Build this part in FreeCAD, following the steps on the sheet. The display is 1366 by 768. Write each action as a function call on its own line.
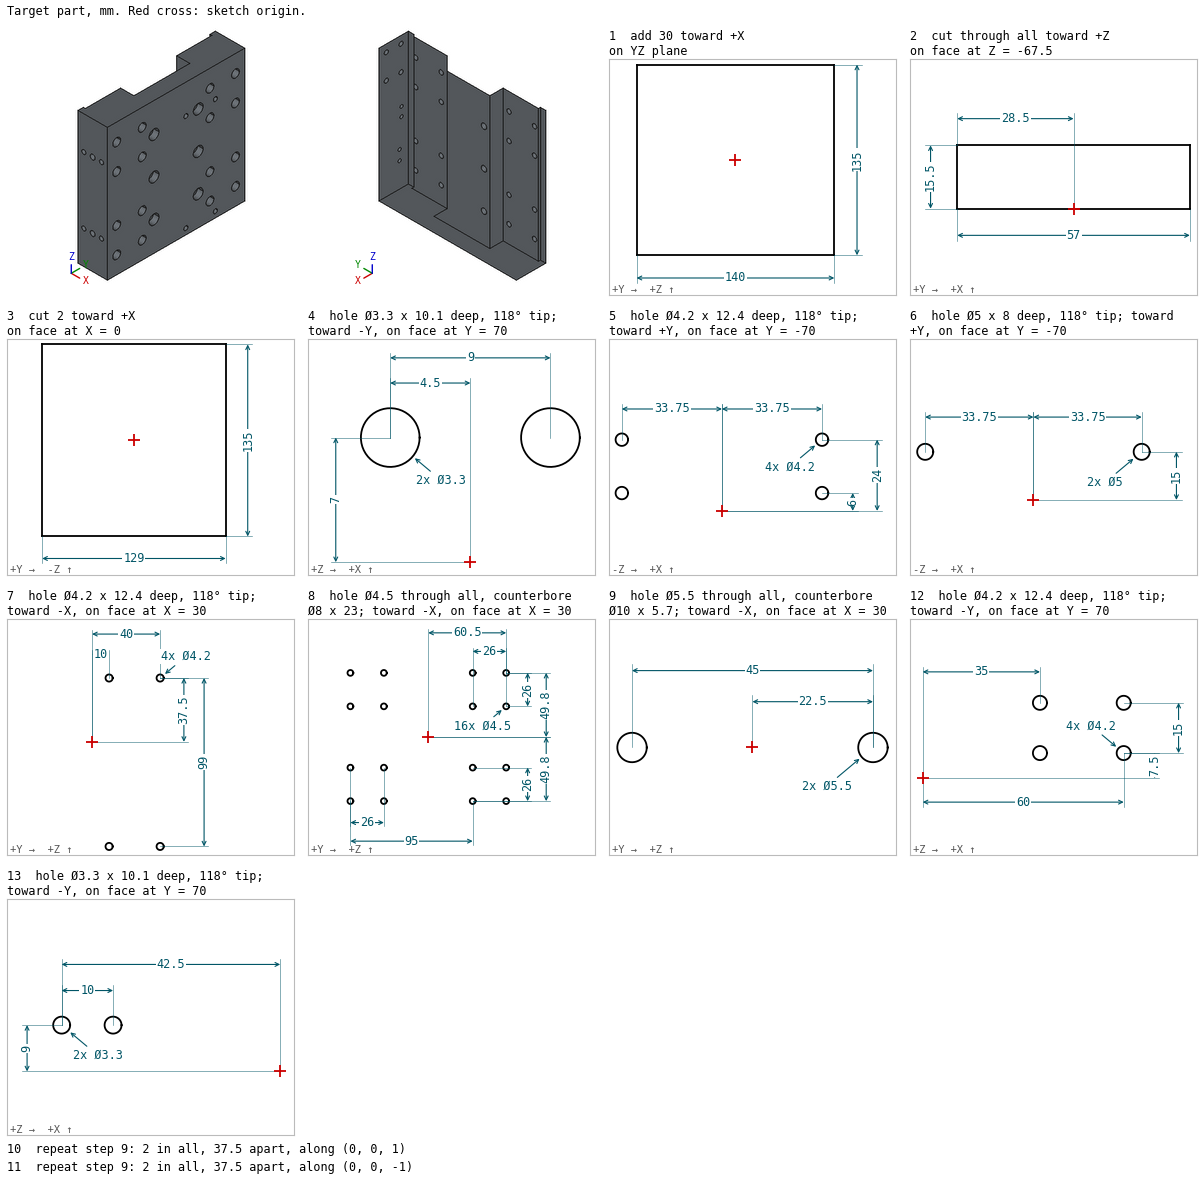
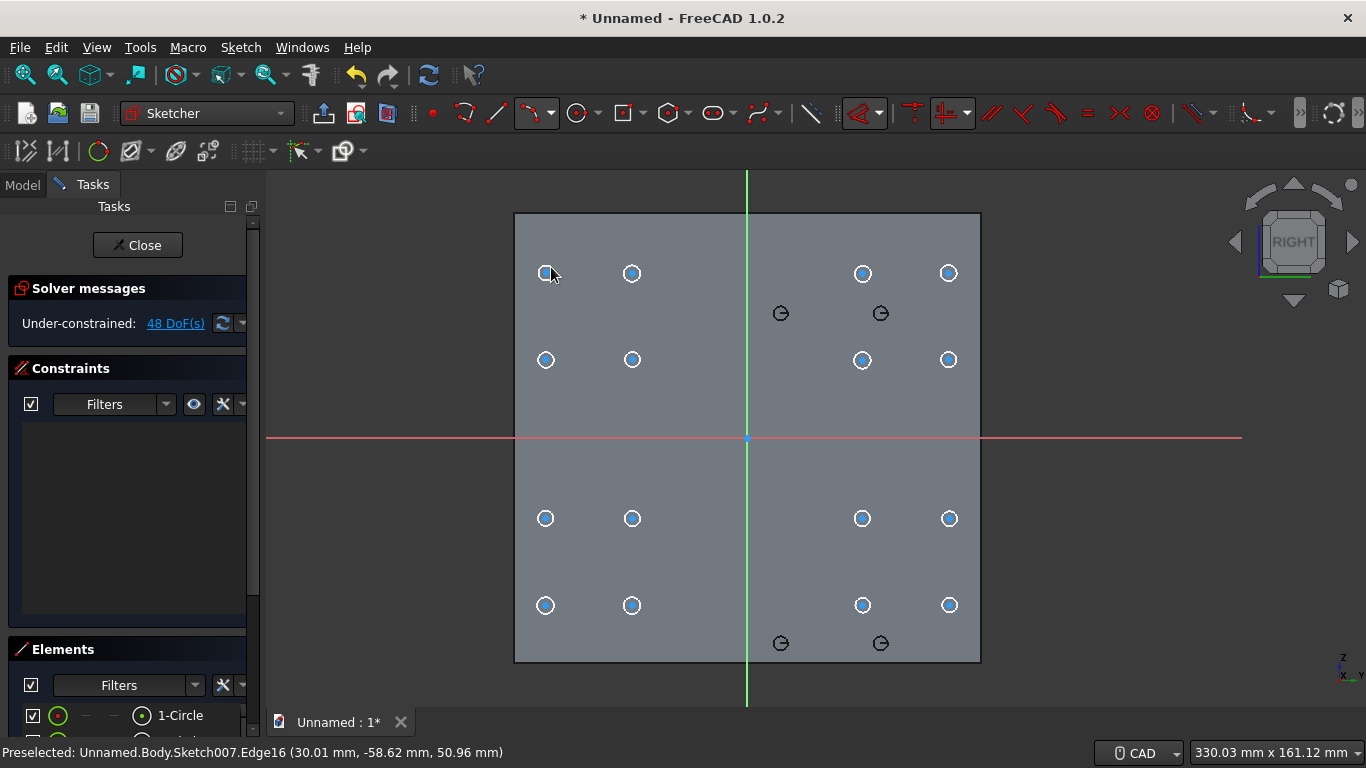
scroll(954, 267, up, 3)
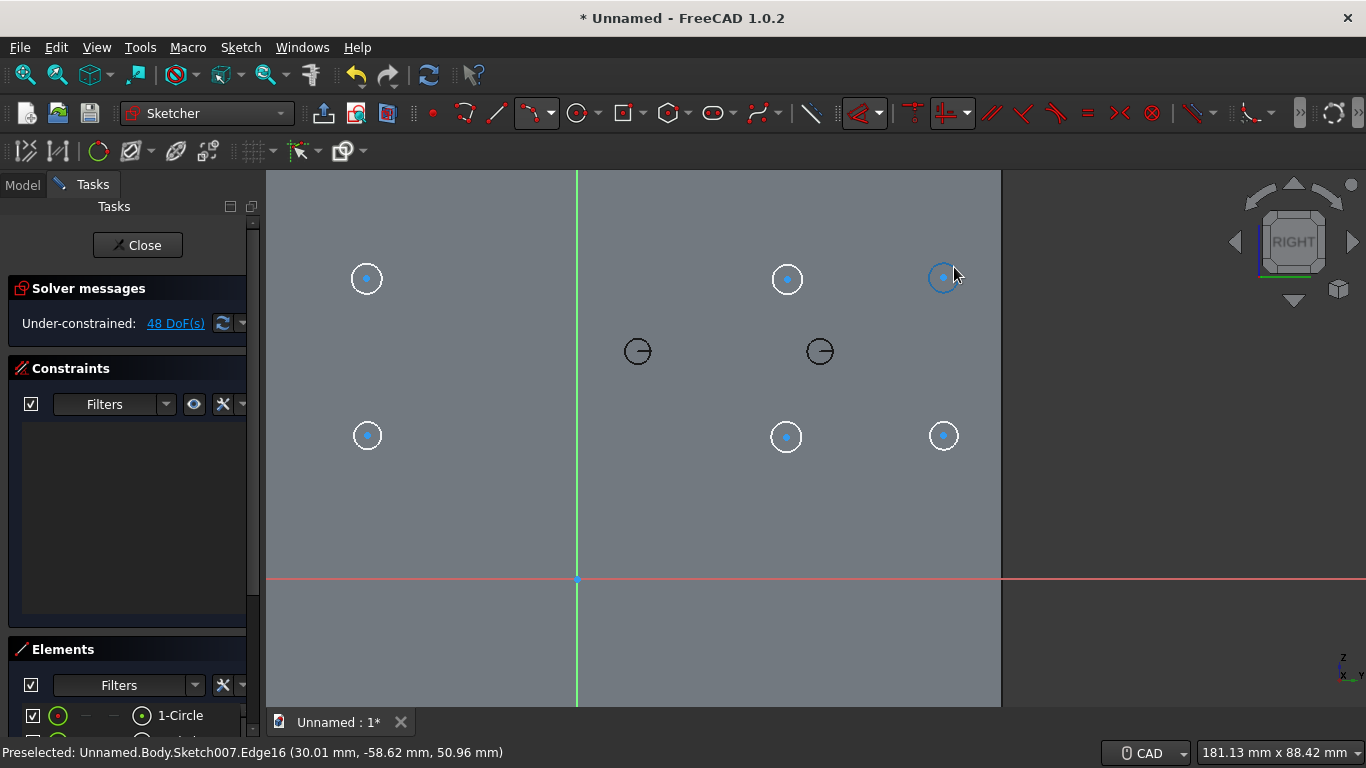
click(954, 268)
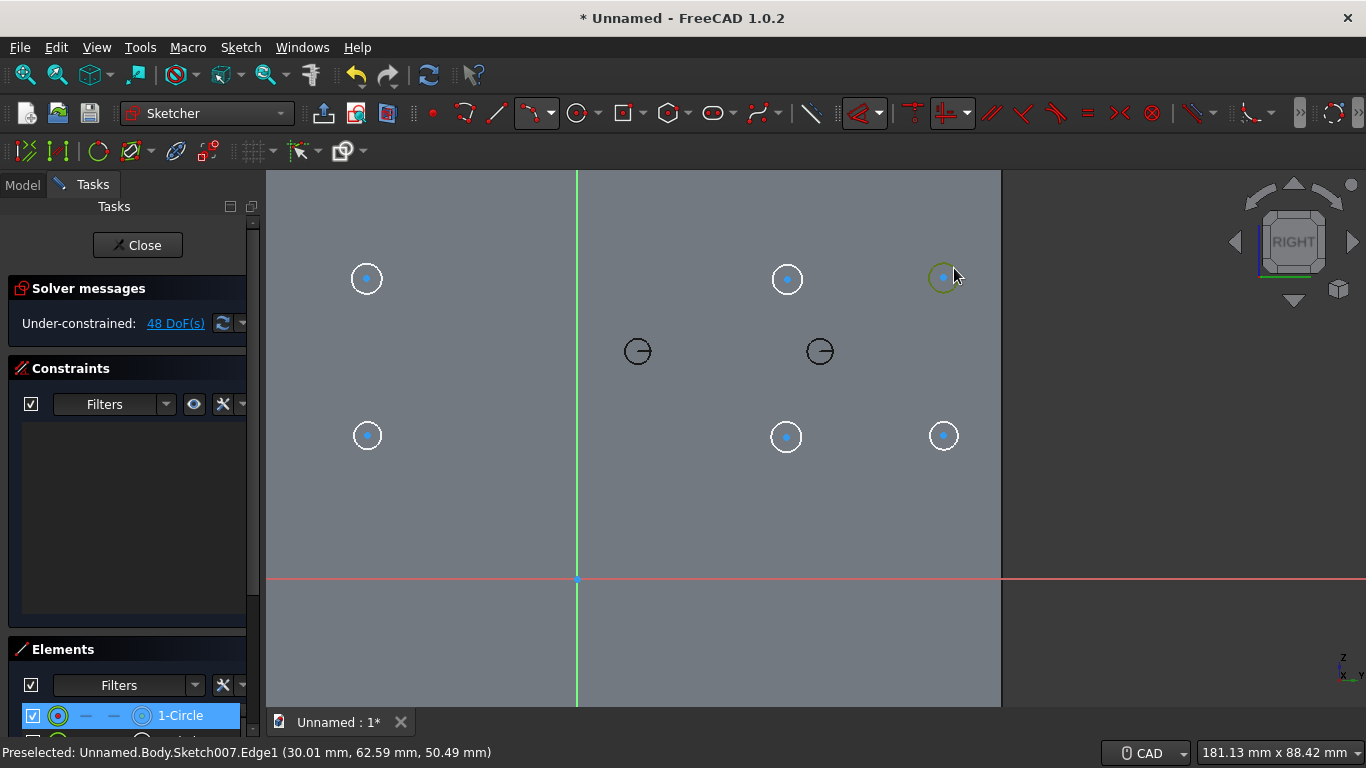
click(954, 426)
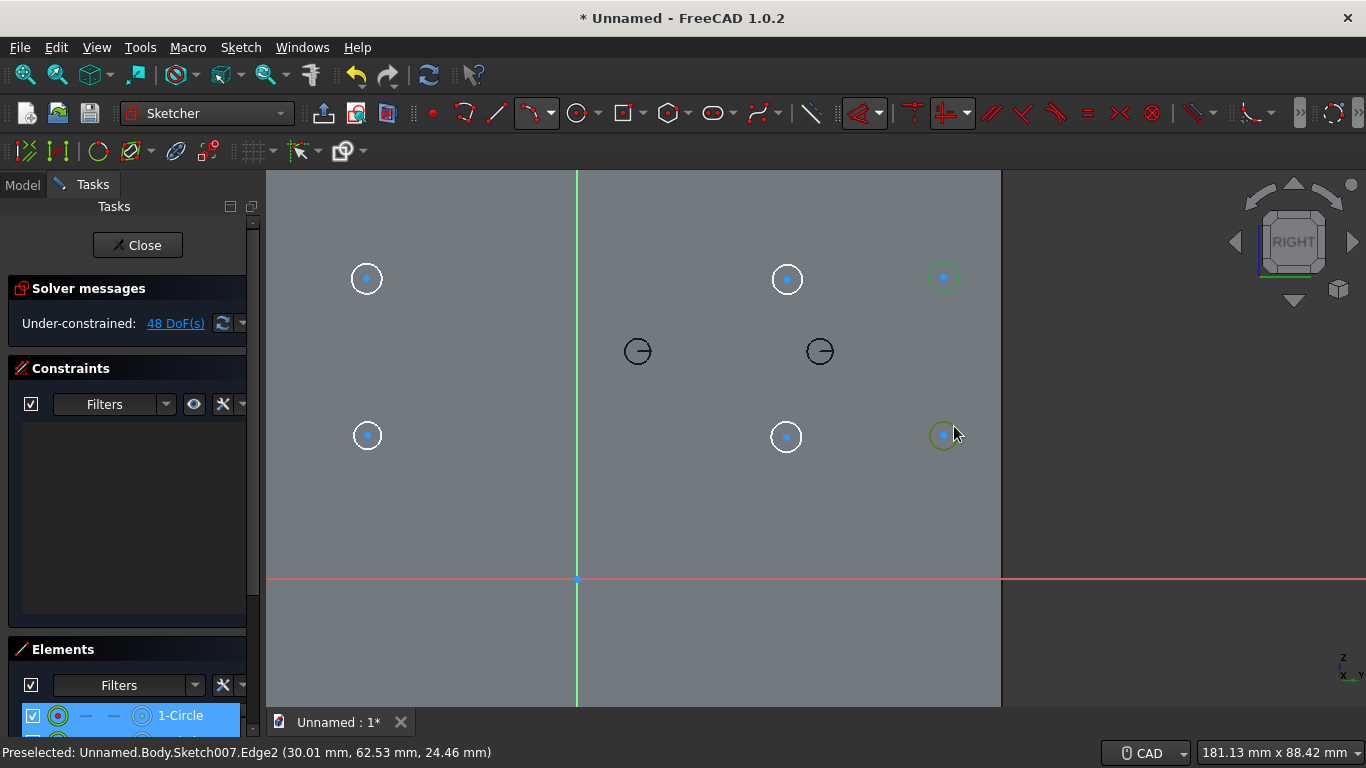
click(797, 426)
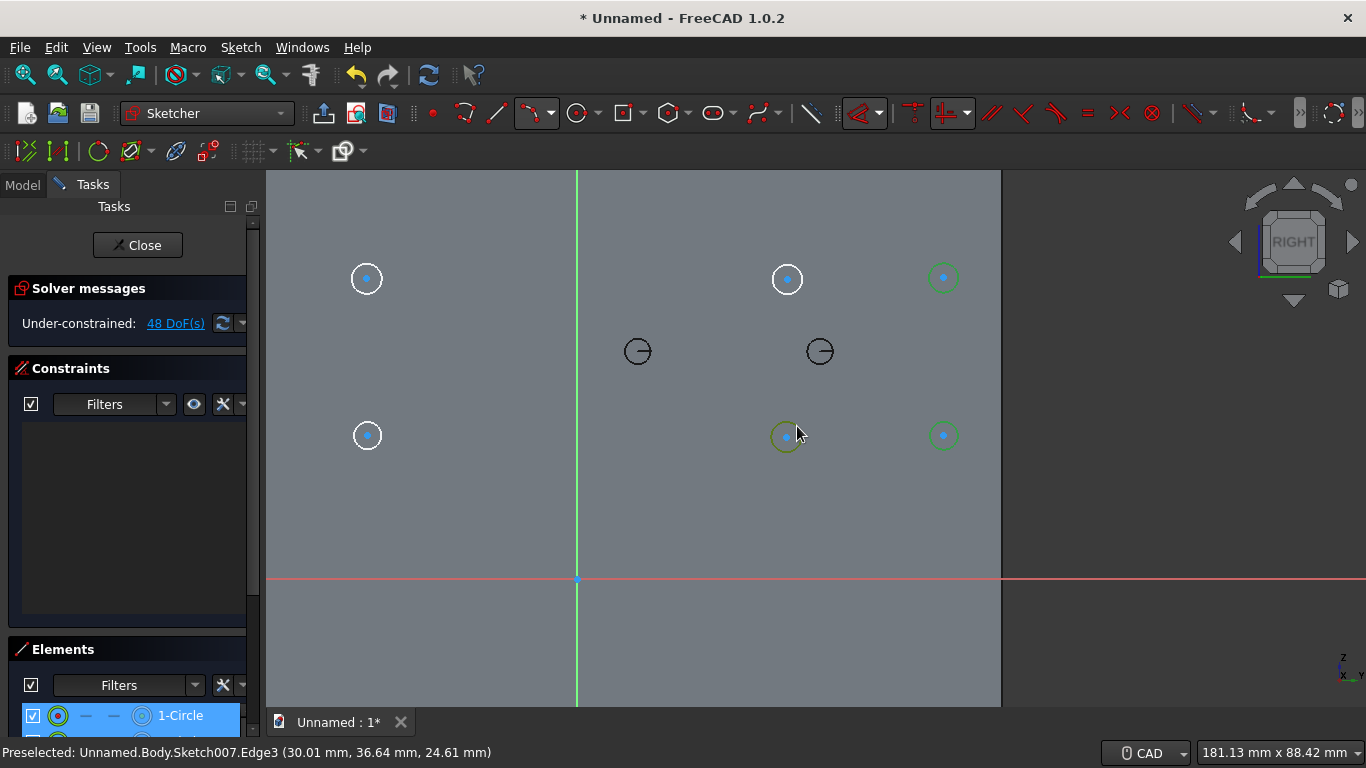
click(798, 269)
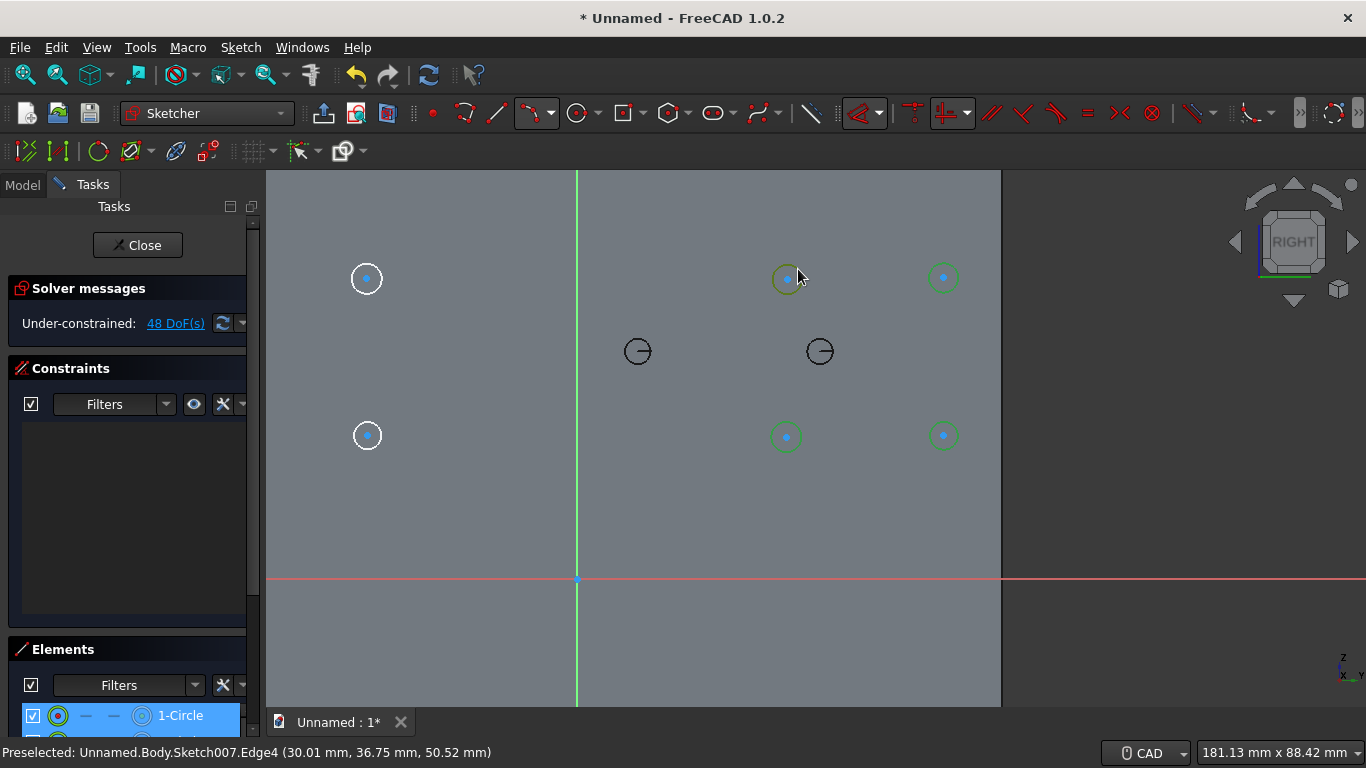
scroll(955, 267, down, 3)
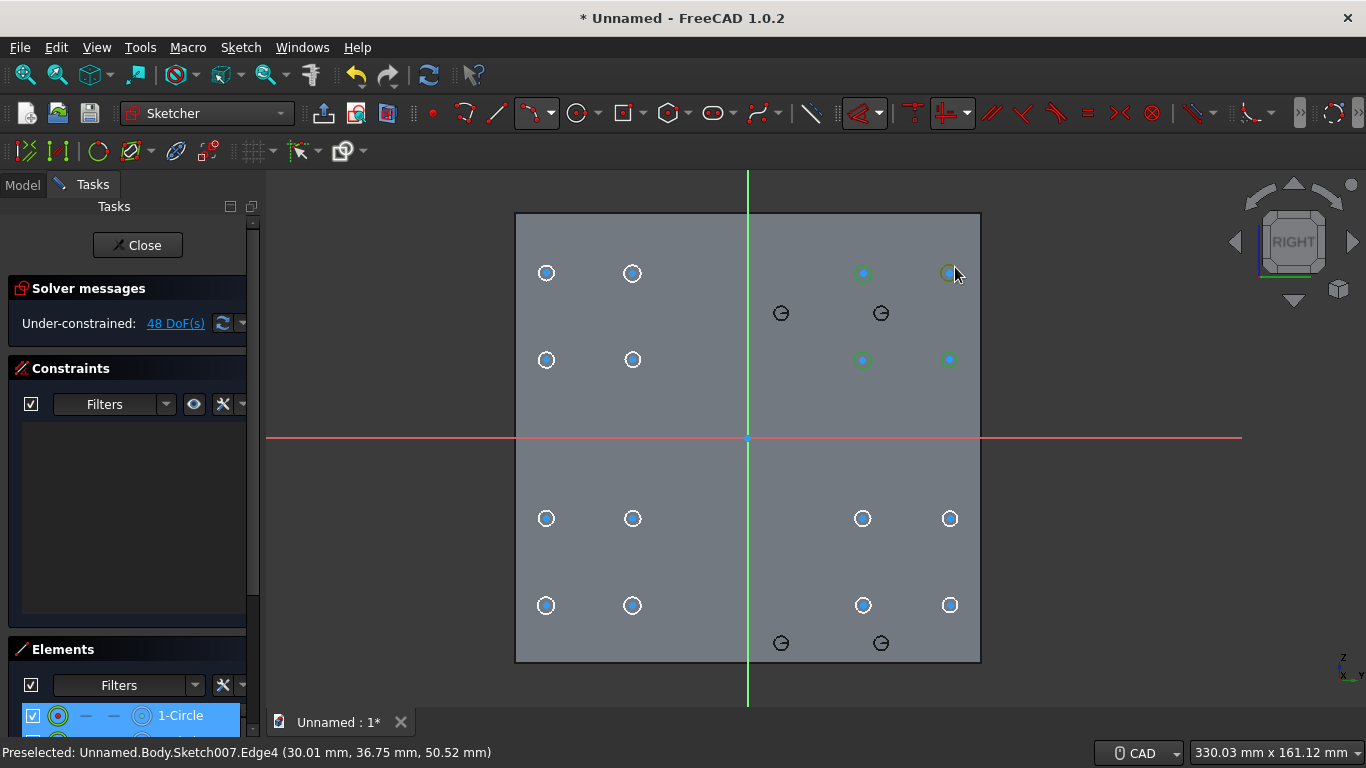
scroll(868, 600, up, 4)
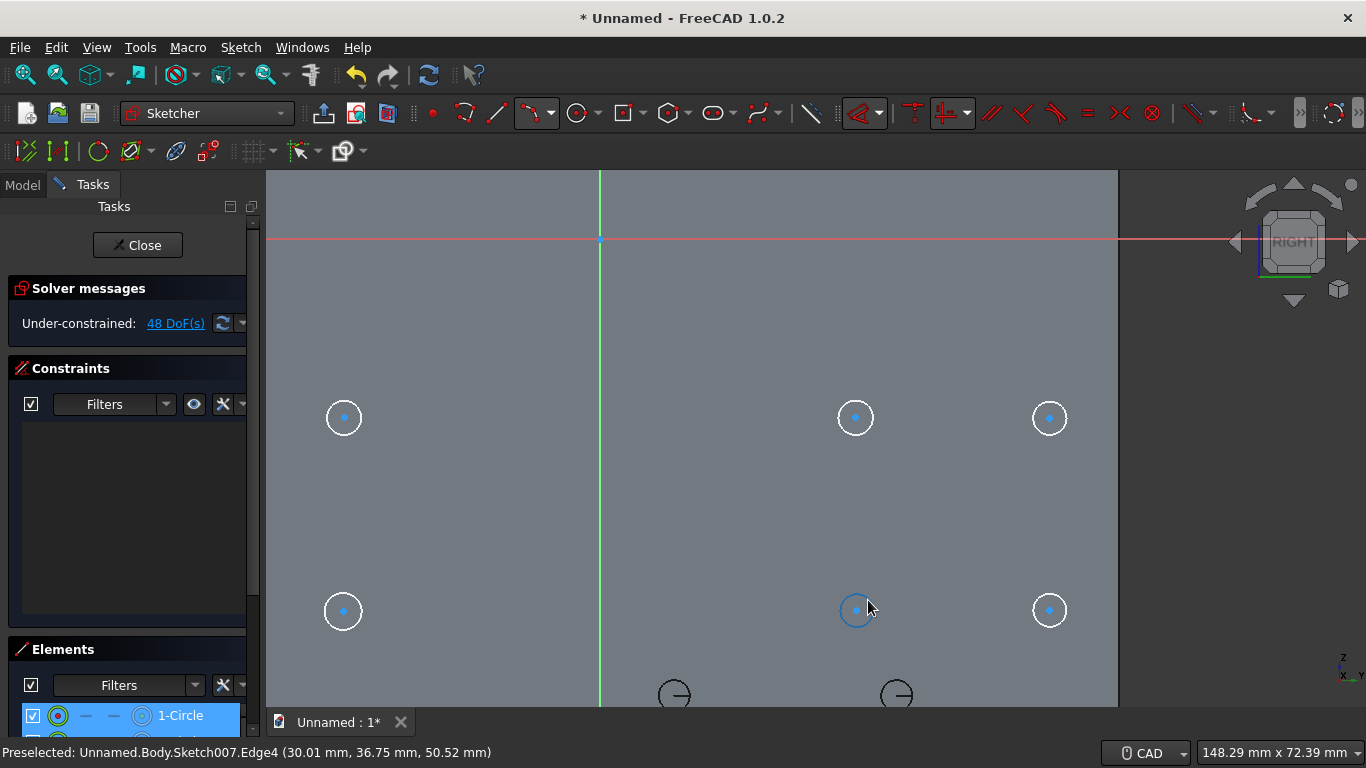
click(868, 599)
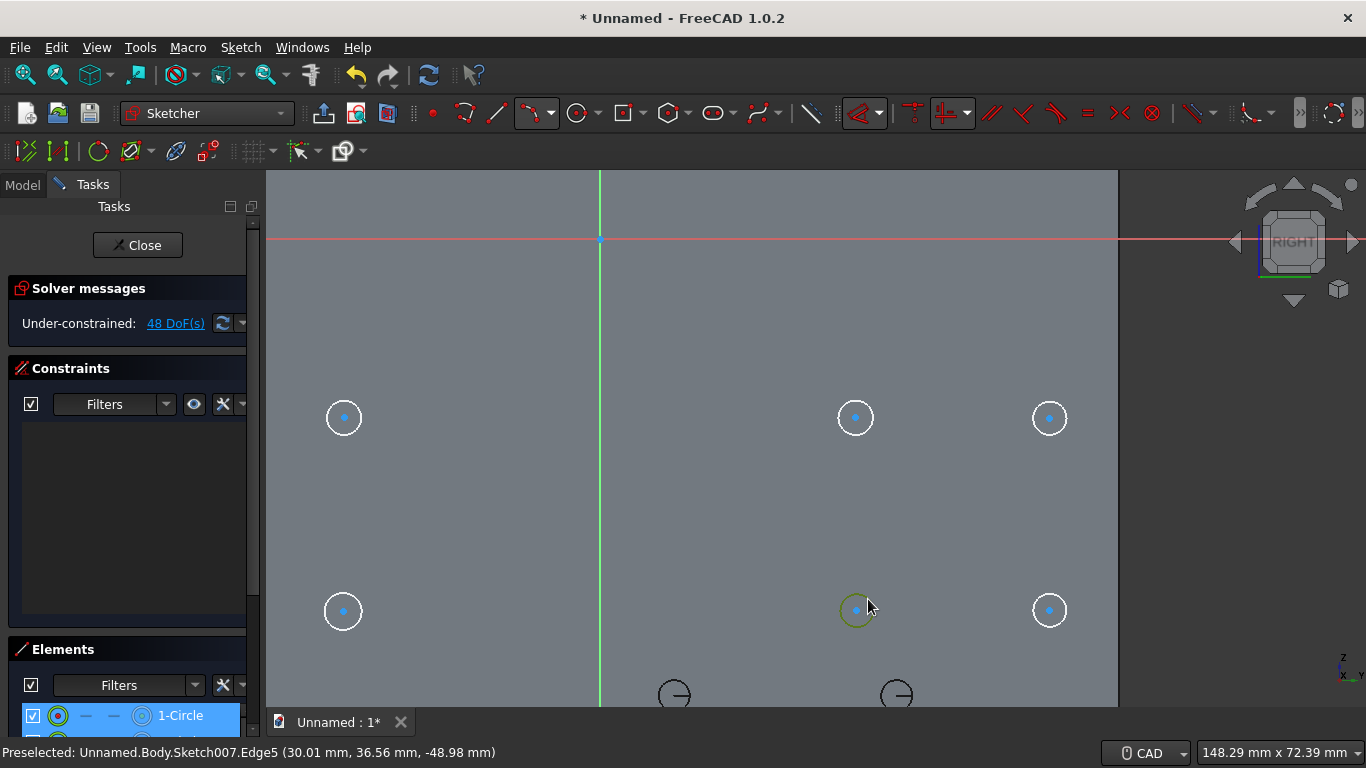
click(868, 405)